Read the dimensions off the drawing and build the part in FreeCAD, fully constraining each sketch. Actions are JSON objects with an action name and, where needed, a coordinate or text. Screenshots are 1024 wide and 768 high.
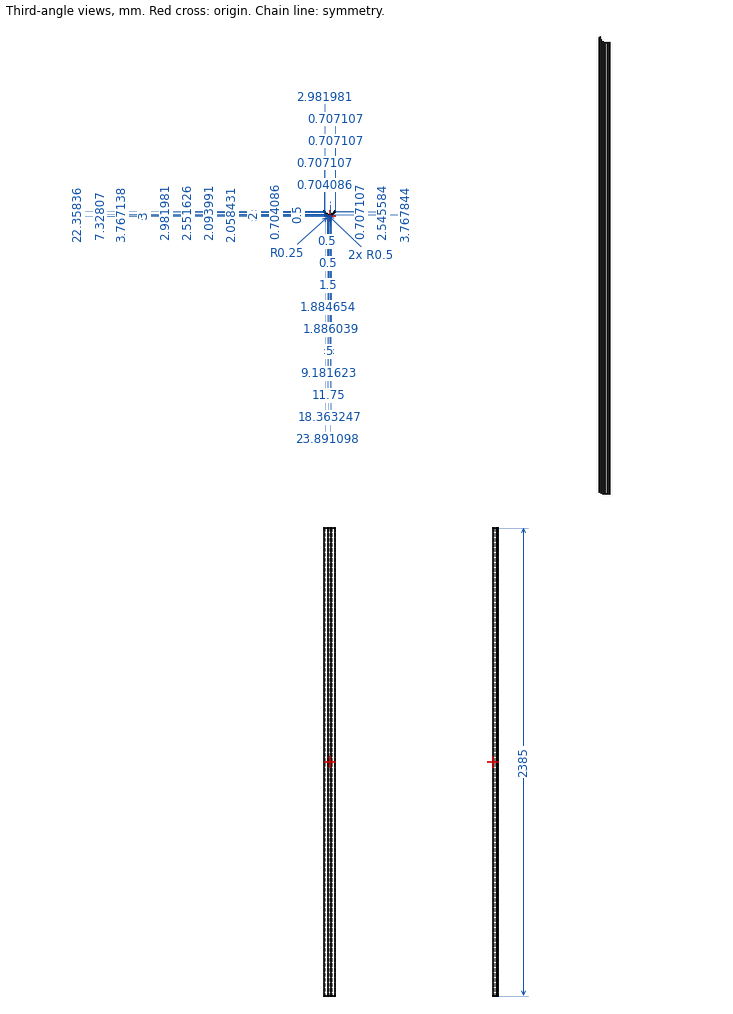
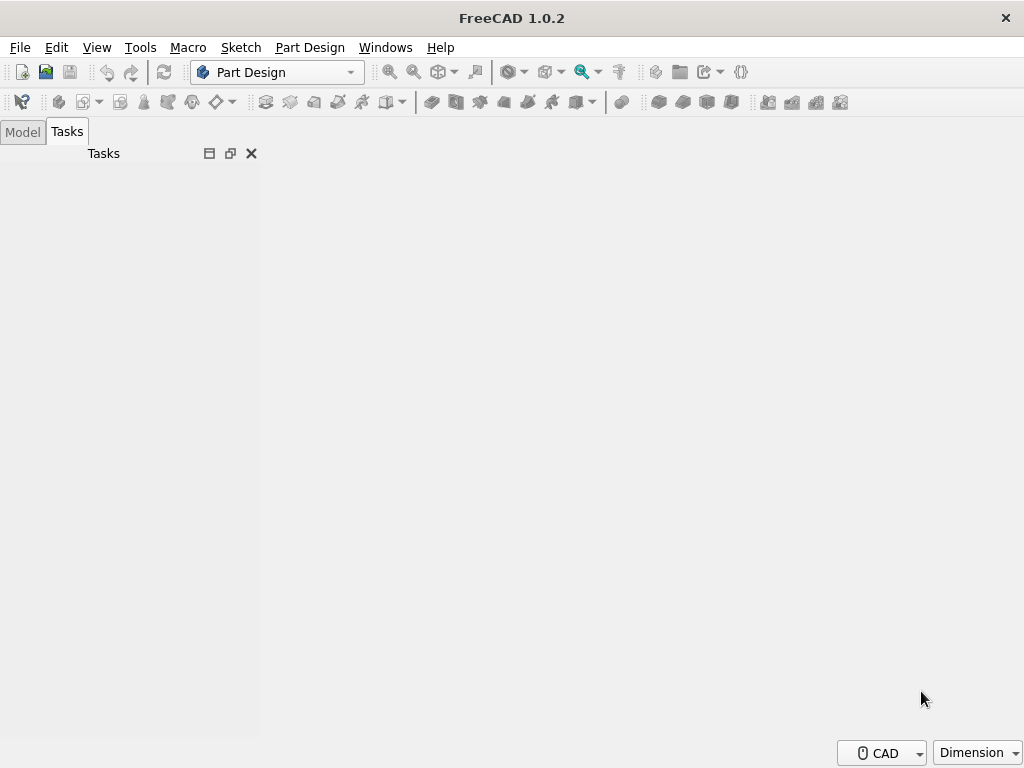
{"action": "key", "text": "ctrl+n"}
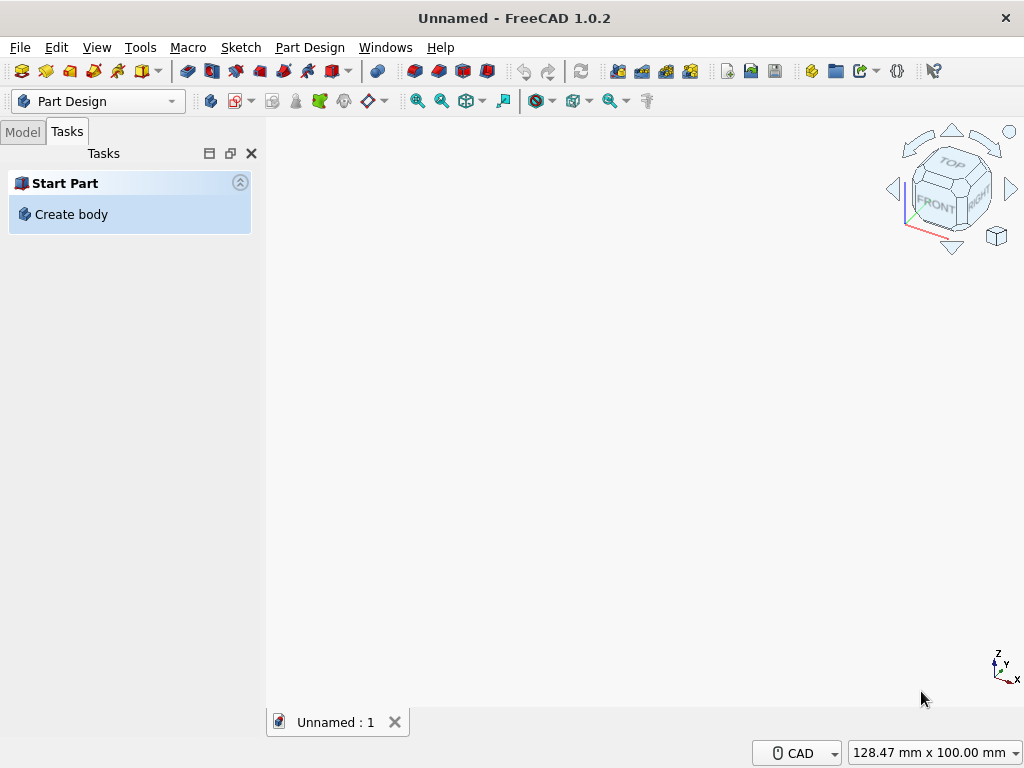
{"action": "left_click", "coordinate": [236, 102]}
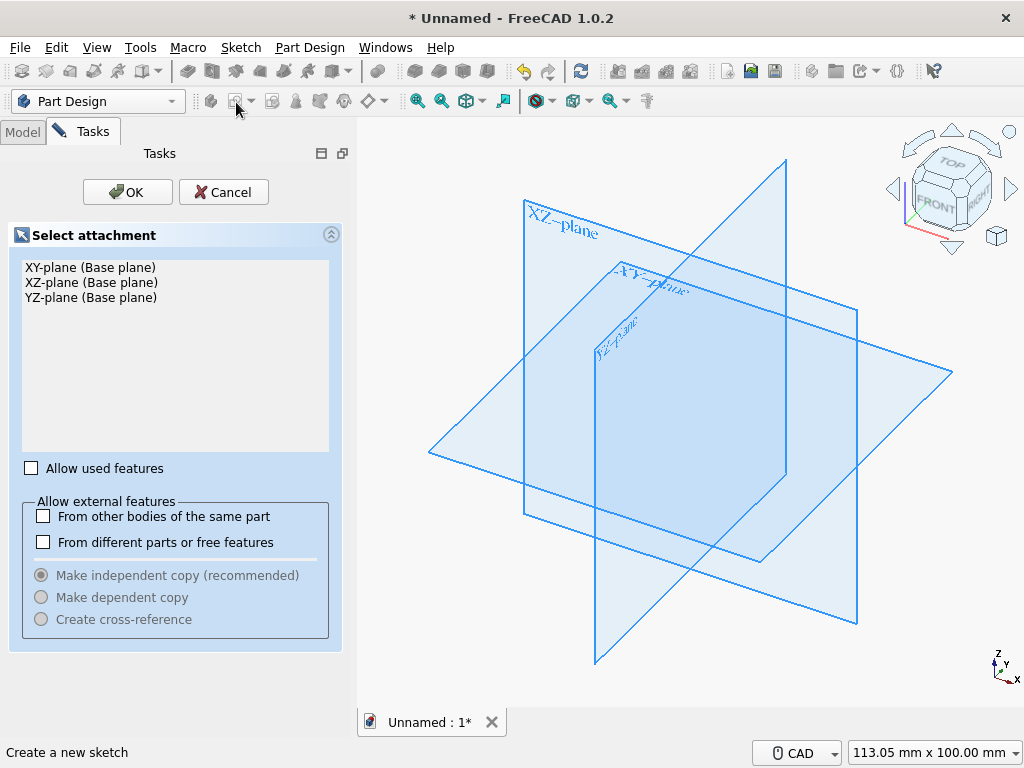
{"action": "left_click", "coordinate": [82, 268]}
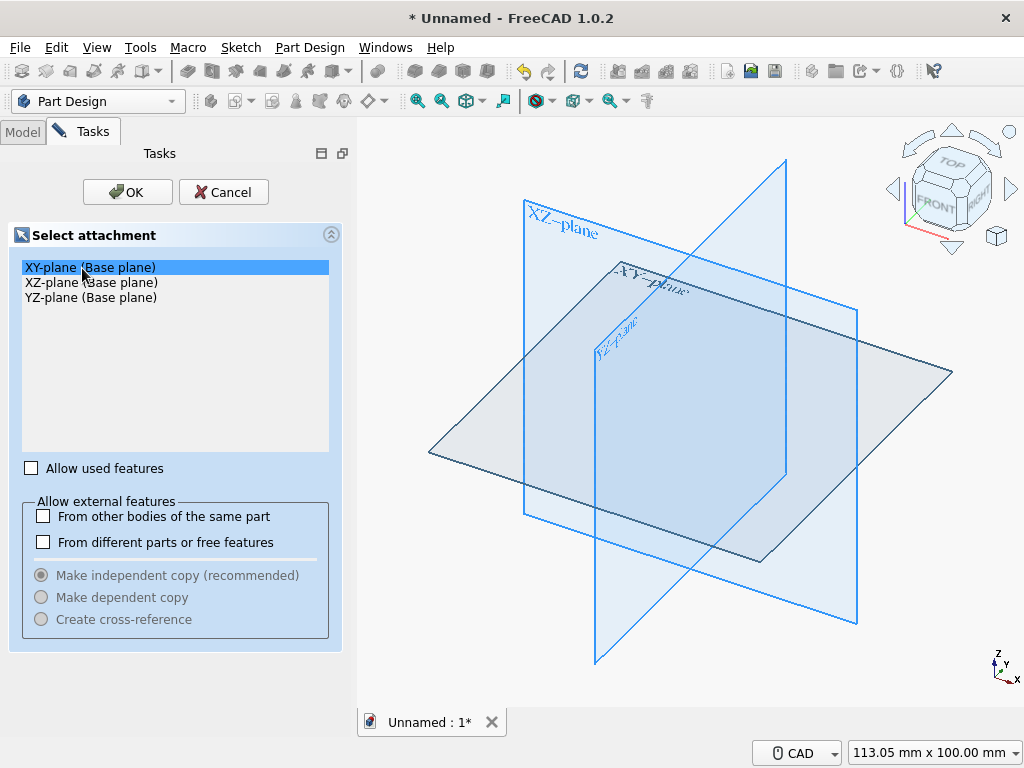
{"action": "left_click", "coordinate": [128, 192]}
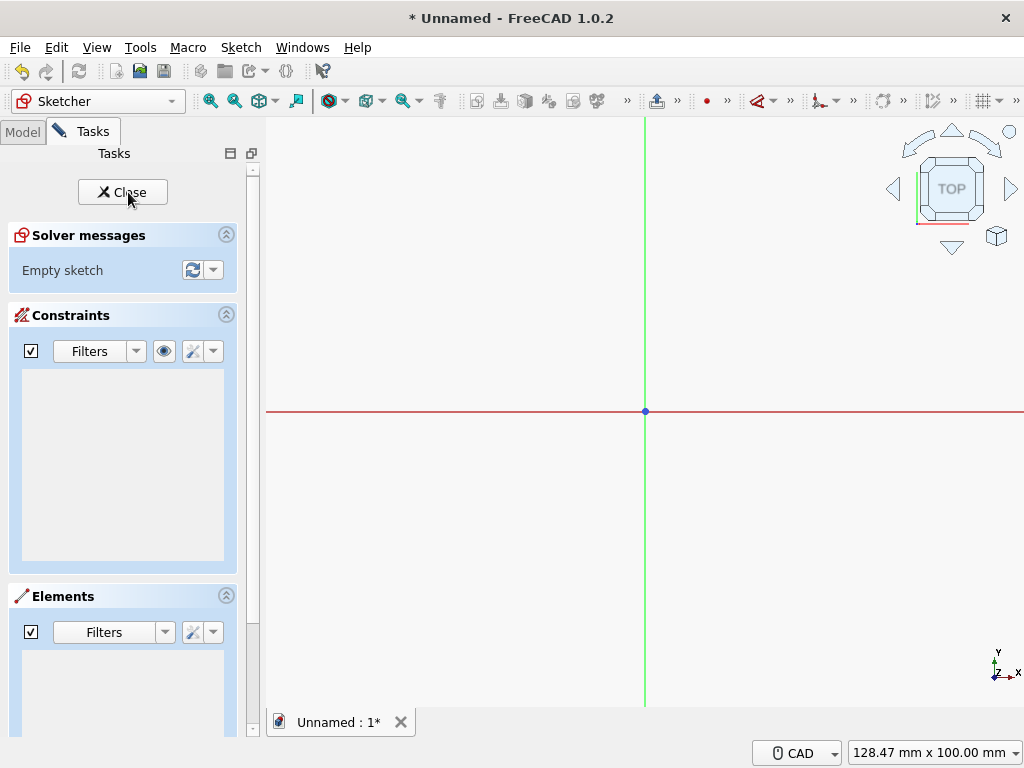
{"action": "key", "text": "g m"}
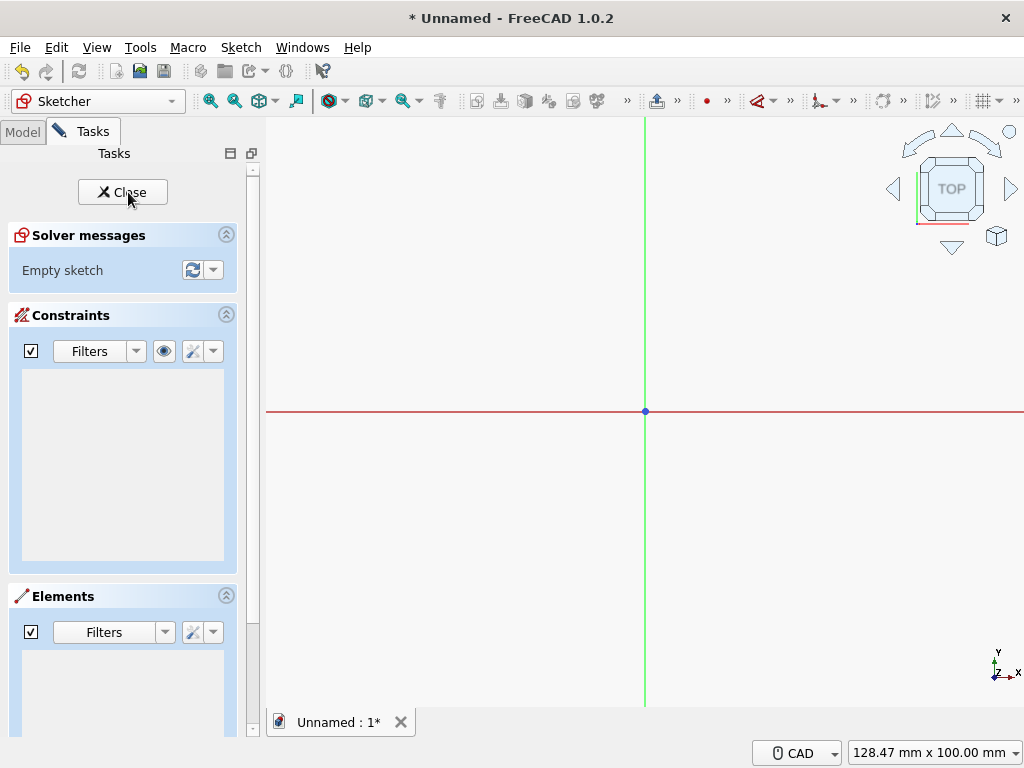
{"action": "scroll", "coordinate": [644, 400], "scroll_direction": "up", "scroll_amount": 12}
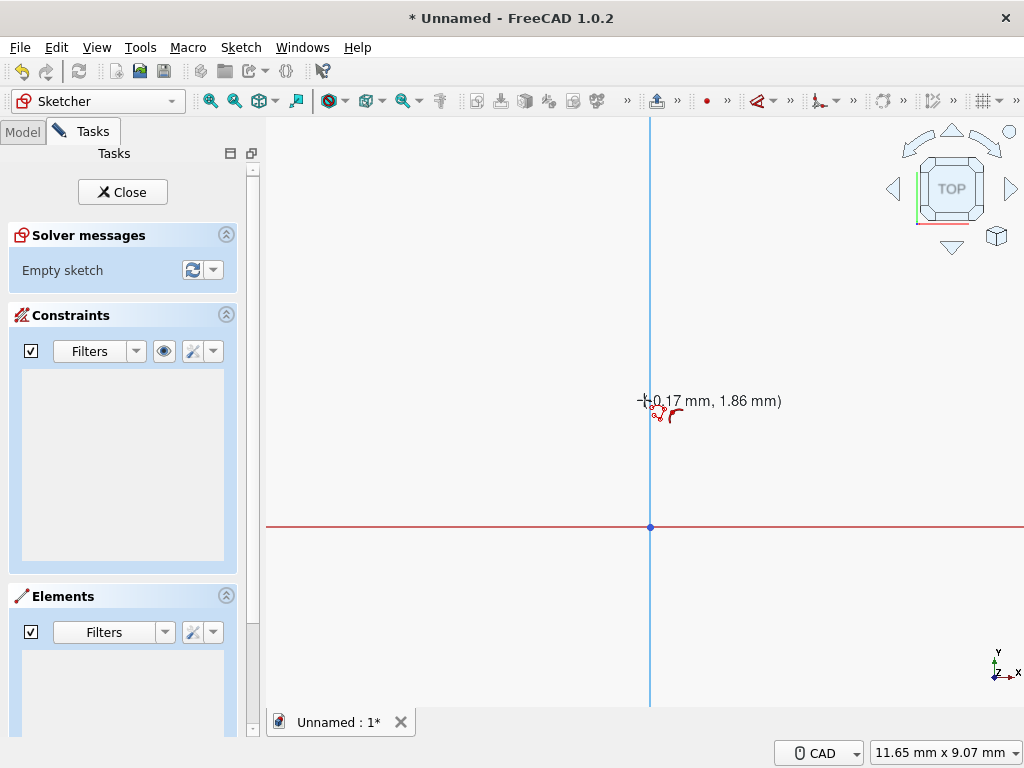
{"action": "left_click", "coordinate": [634, 397]}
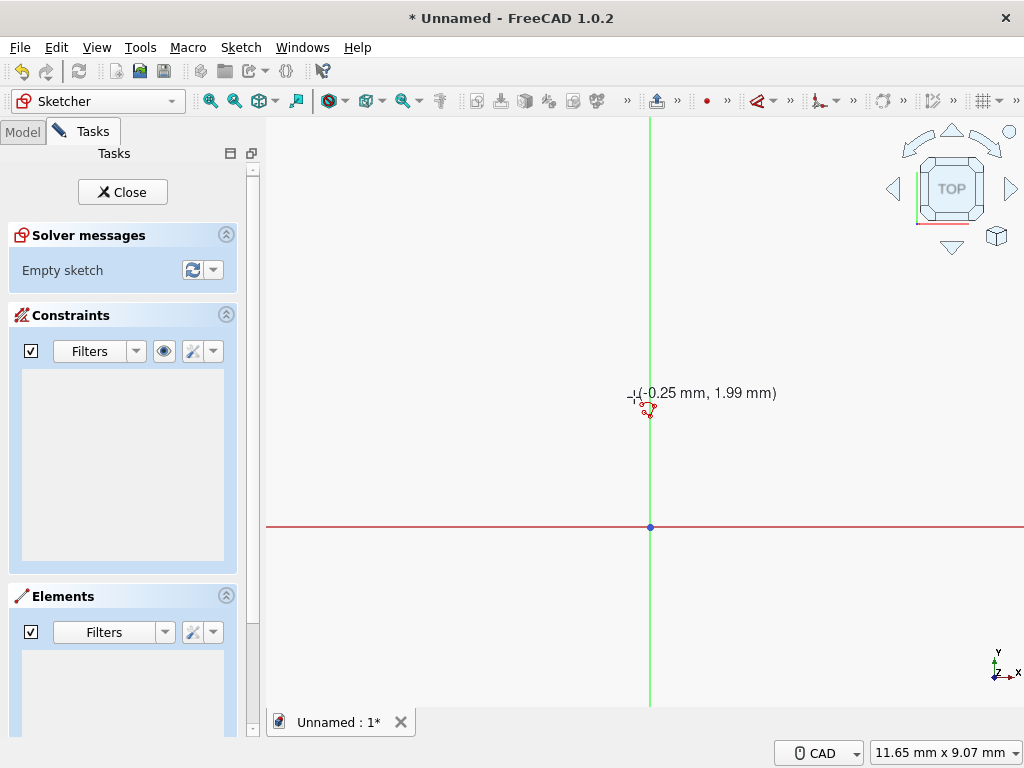
{"action": "scroll", "coordinate": [567, 488], "scroll_direction": "down", "scroll_amount": 11}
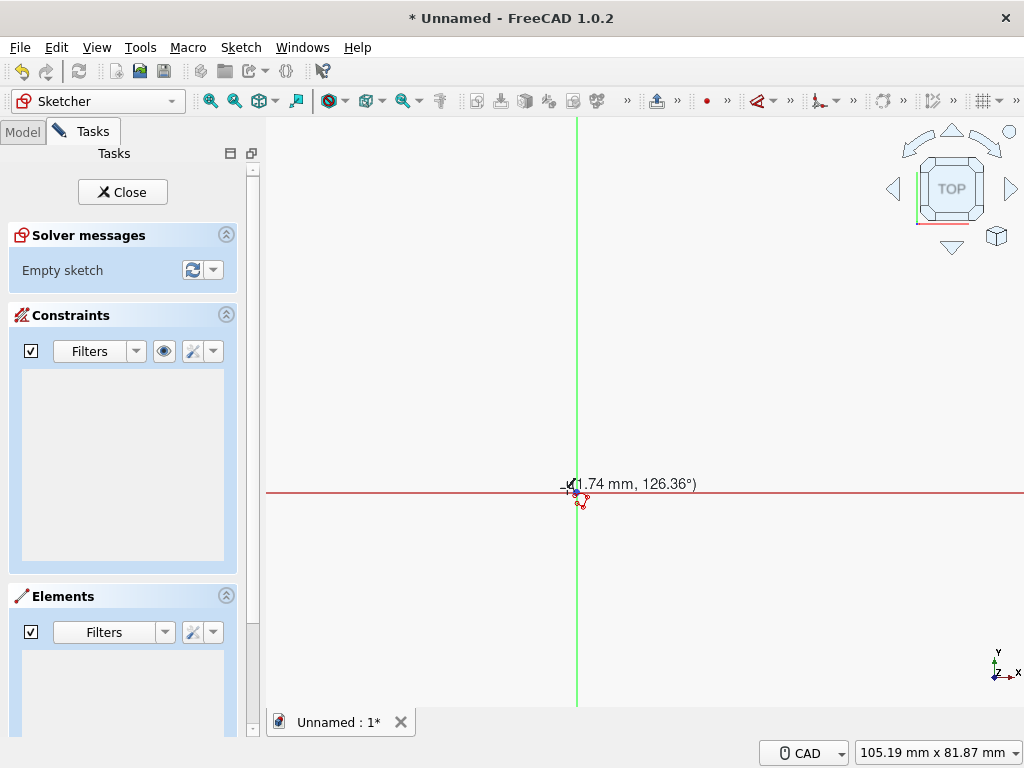
{"action": "left_click", "coordinate": [539, 478]}
{"action": "left_click", "coordinate": [539, 457]}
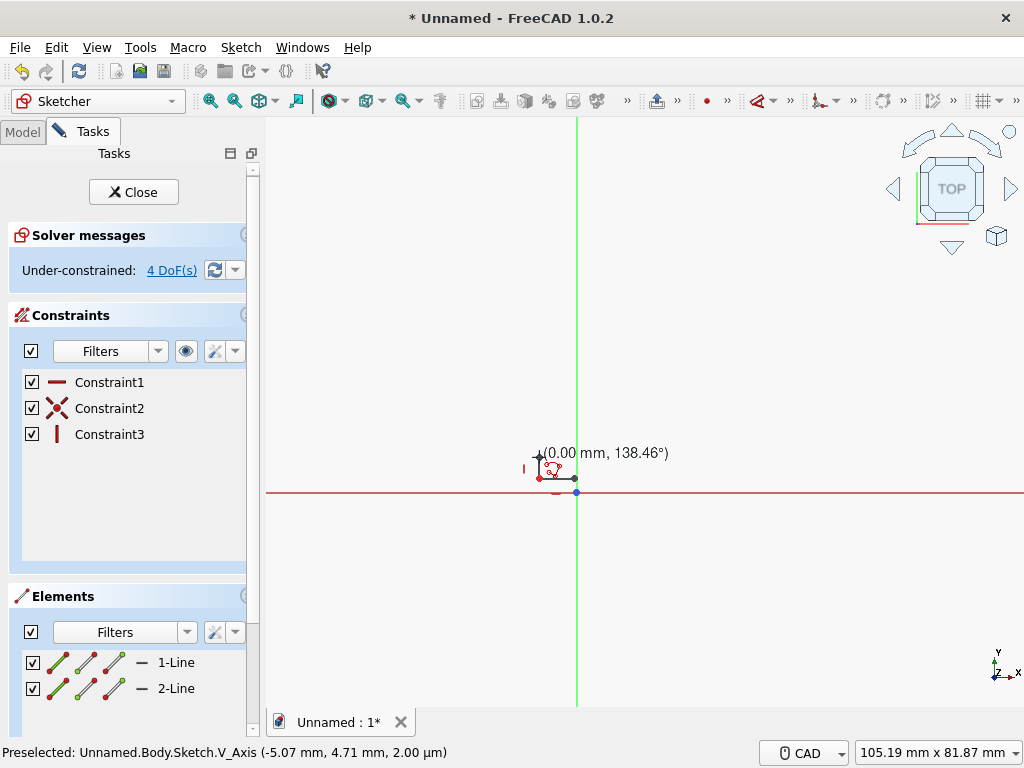
{"action": "scroll", "coordinate": [528, 457], "scroll_direction": "up", "scroll_amount": 2}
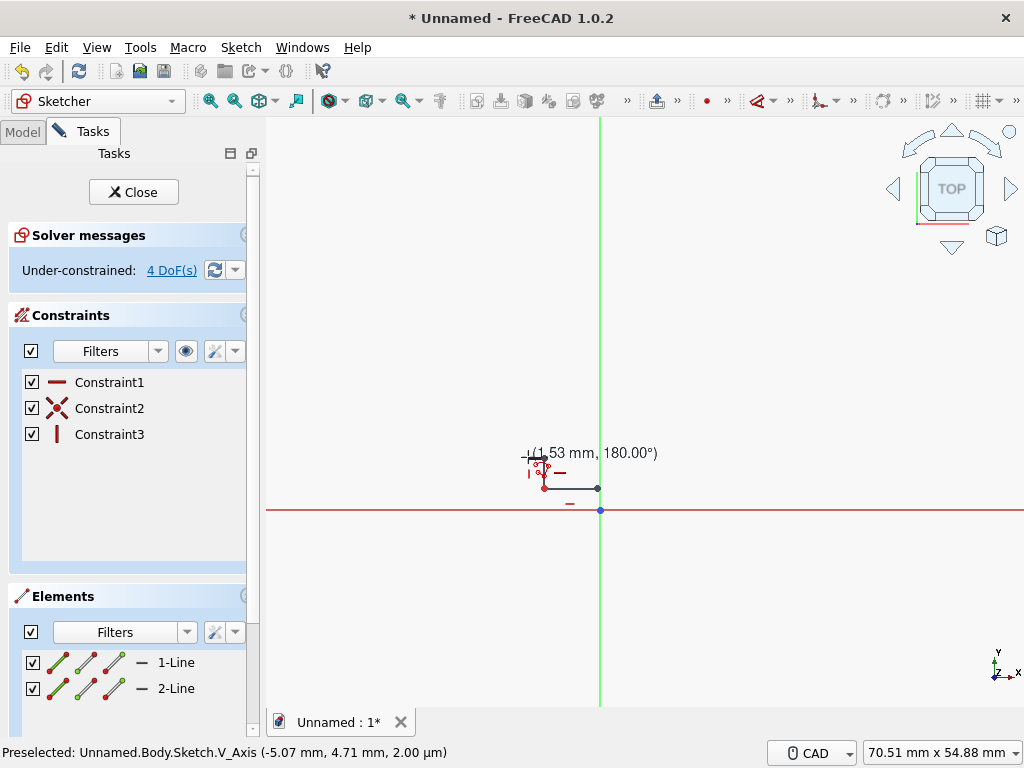
{"action": "left_click", "coordinate": [528, 457]}
{"action": "left_click", "coordinate": [528, 489]}
{"action": "left_click", "coordinate": [507, 489]}
{"action": "left_click", "coordinate": [474, 455]}
{"action": "left_click", "coordinate": [474, 415]}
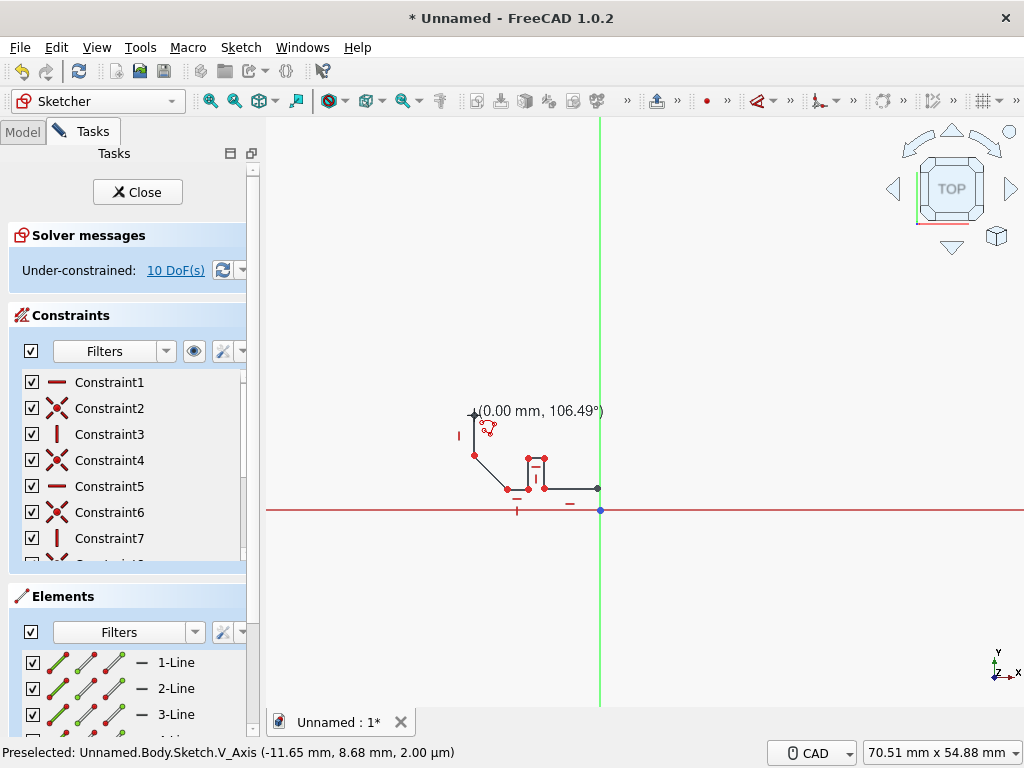
{"action": "scroll", "coordinate": [469, 409], "scroll_direction": "up", "scroll_amount": 4}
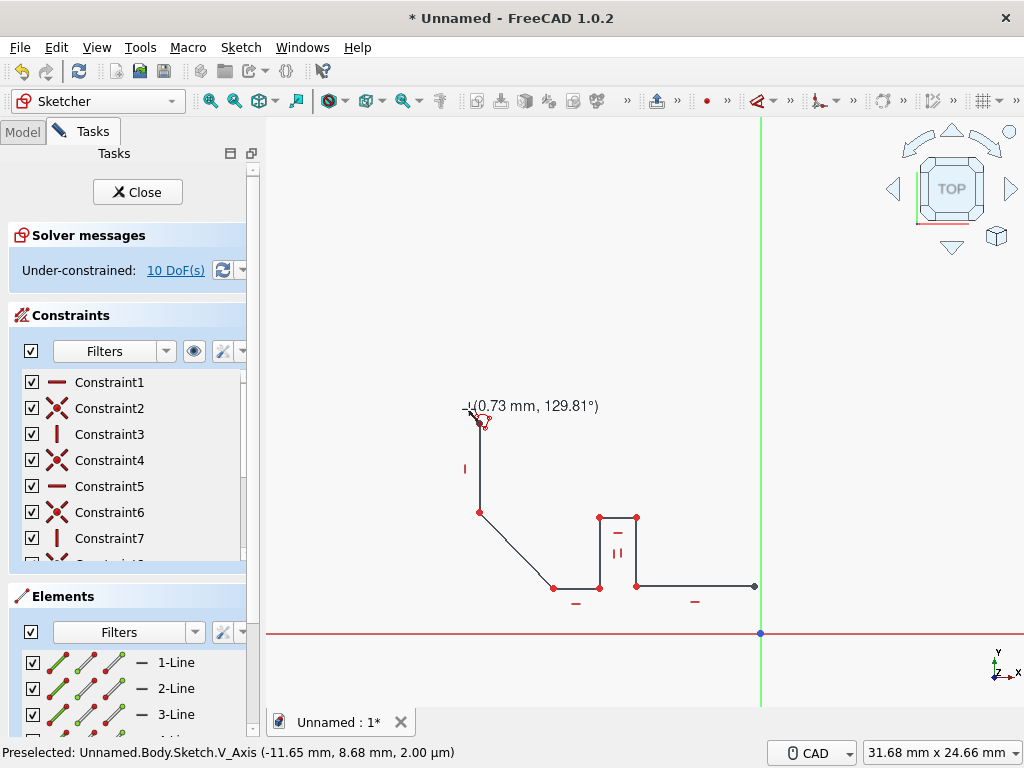
{"action": "left_click", "coordinate": [468, 409]}